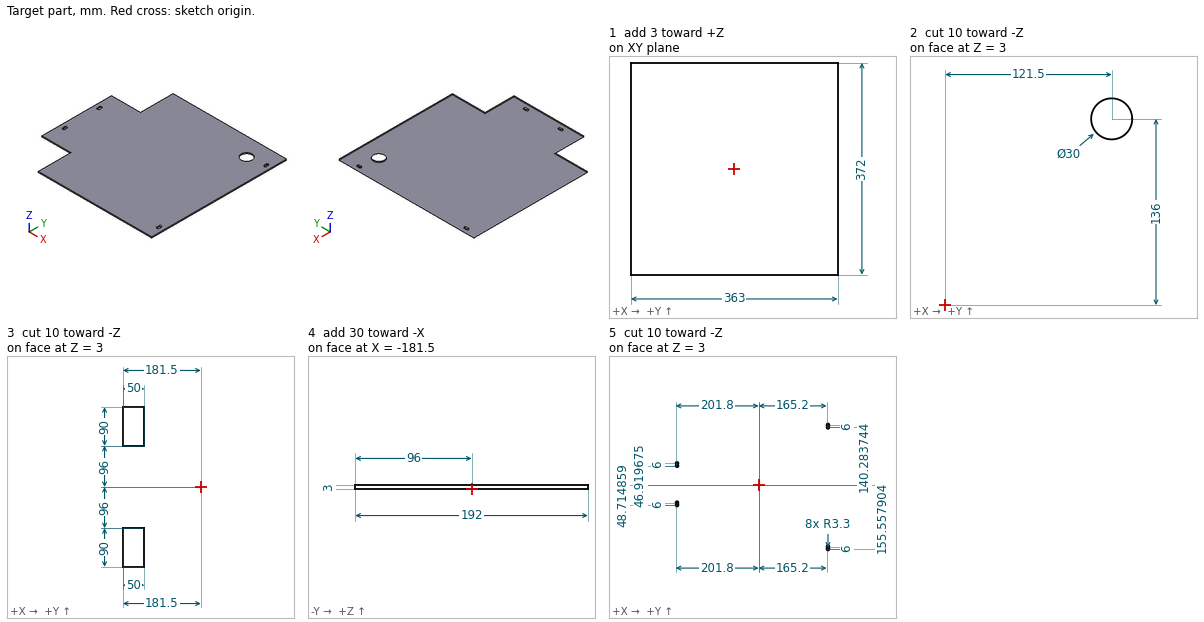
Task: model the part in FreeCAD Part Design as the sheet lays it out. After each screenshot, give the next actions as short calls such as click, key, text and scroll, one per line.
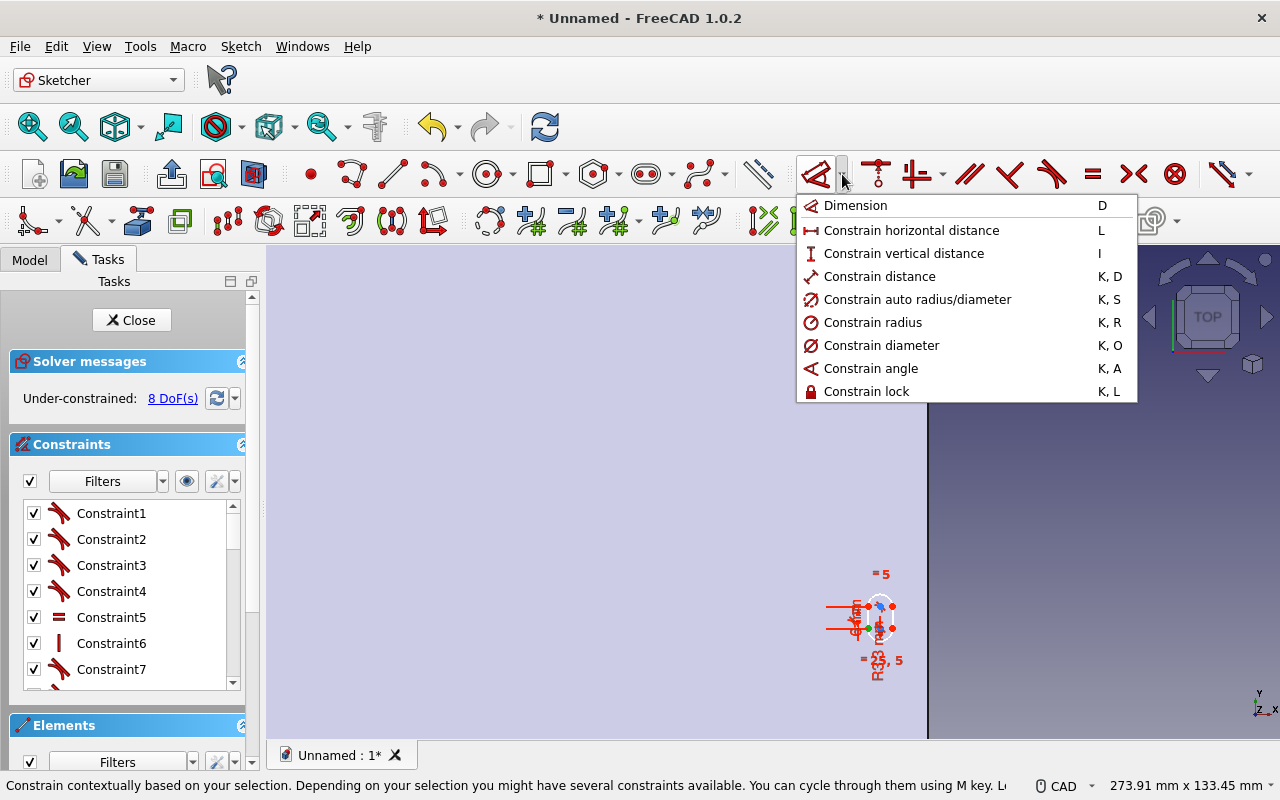
click(967, 230)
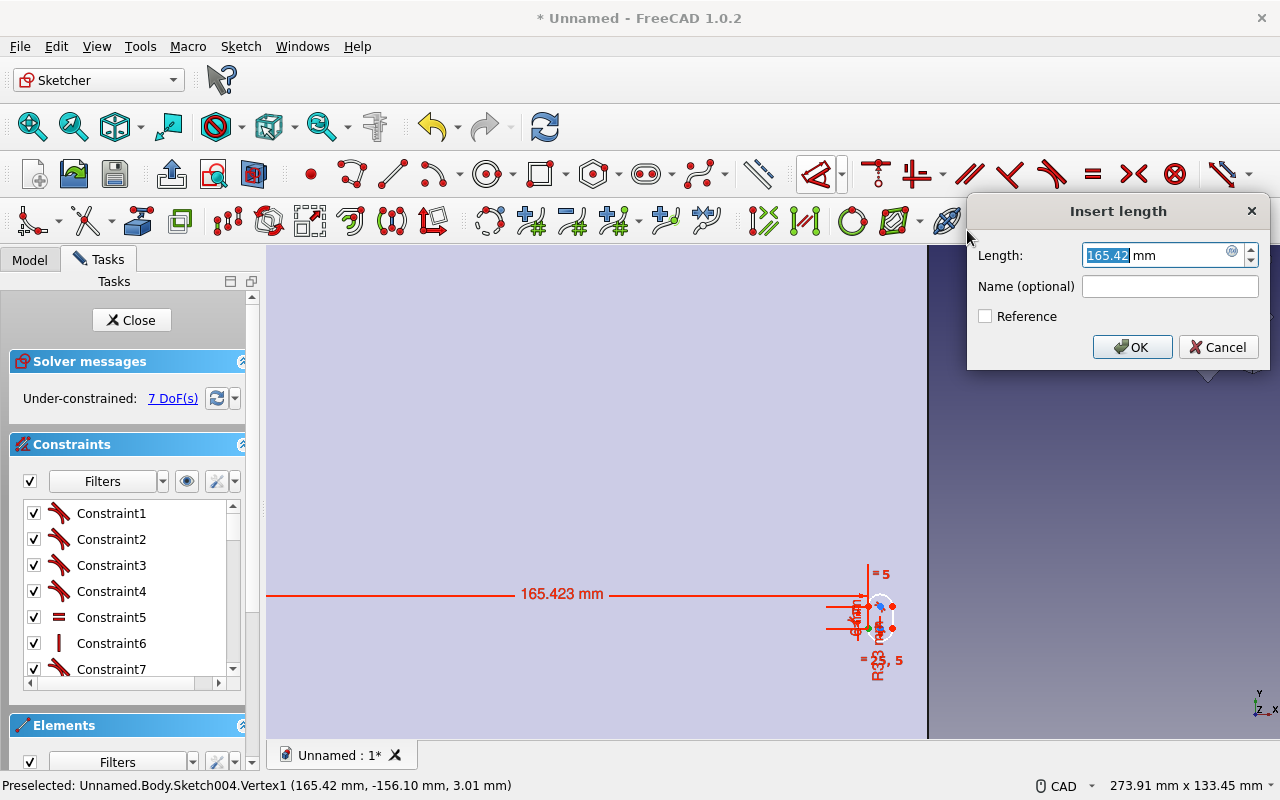
text(165.2)
key(Return)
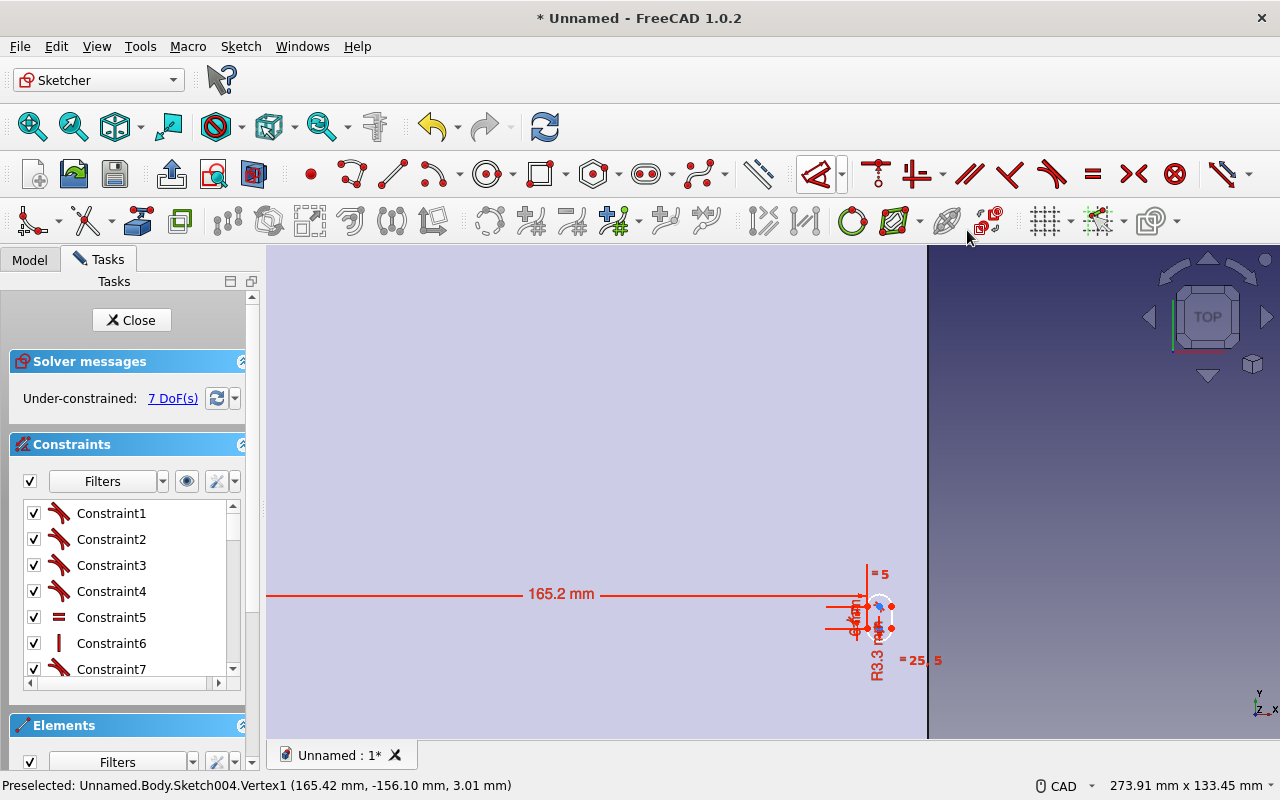
scroll(870, 631, down, 7)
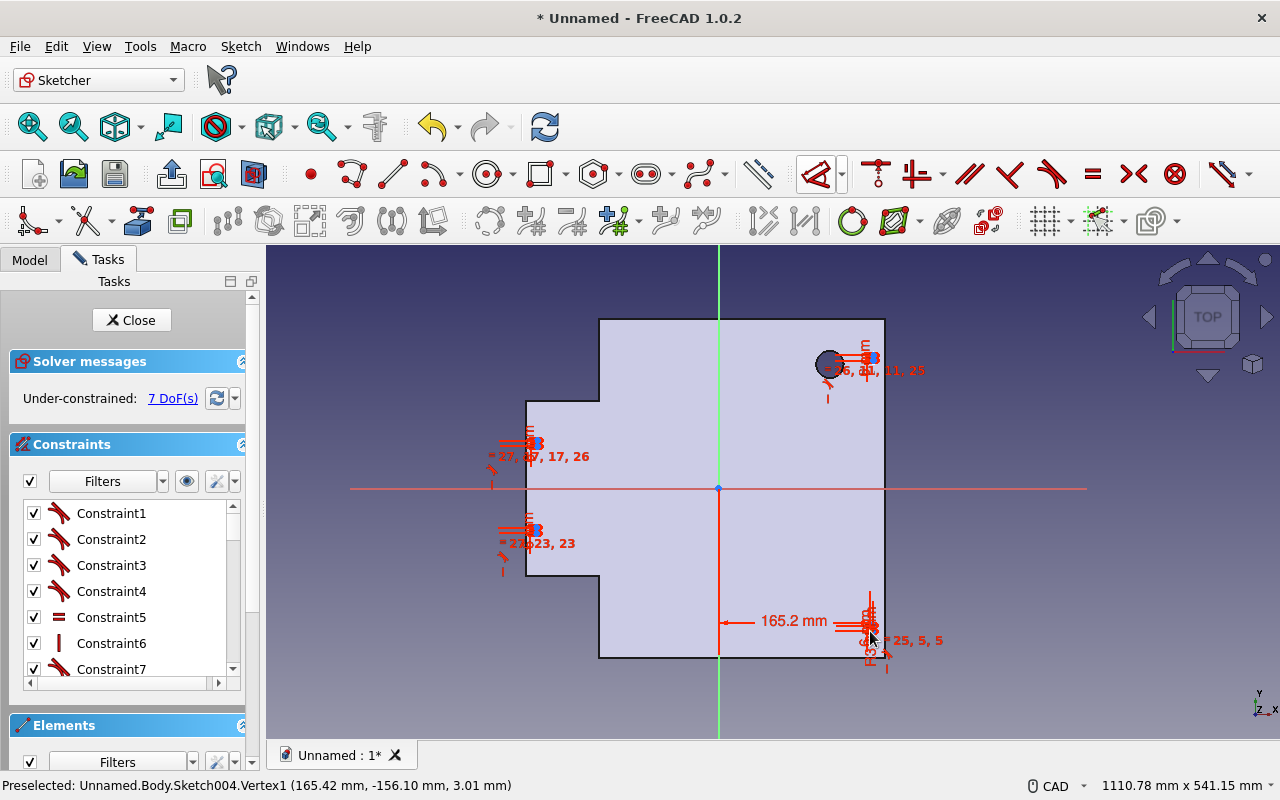
scroll(870, 361, up, 7)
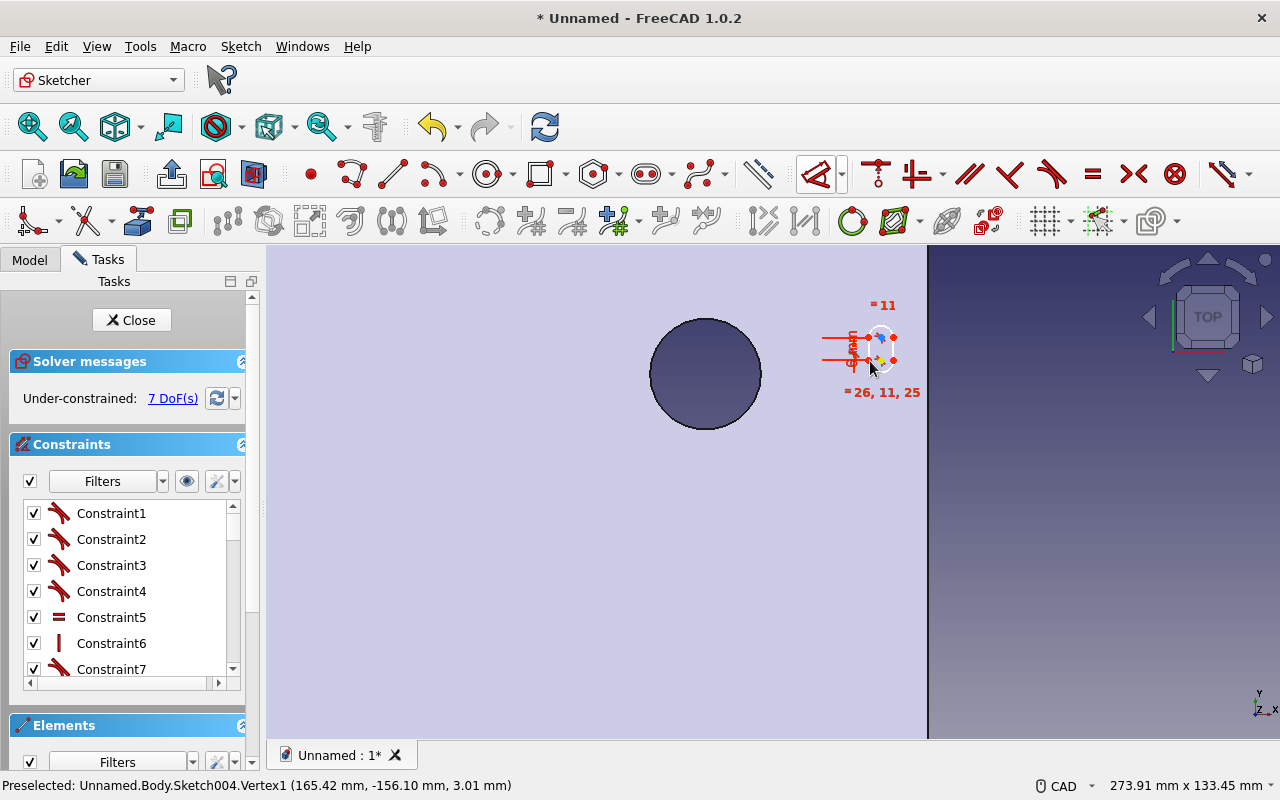
click(869, 360)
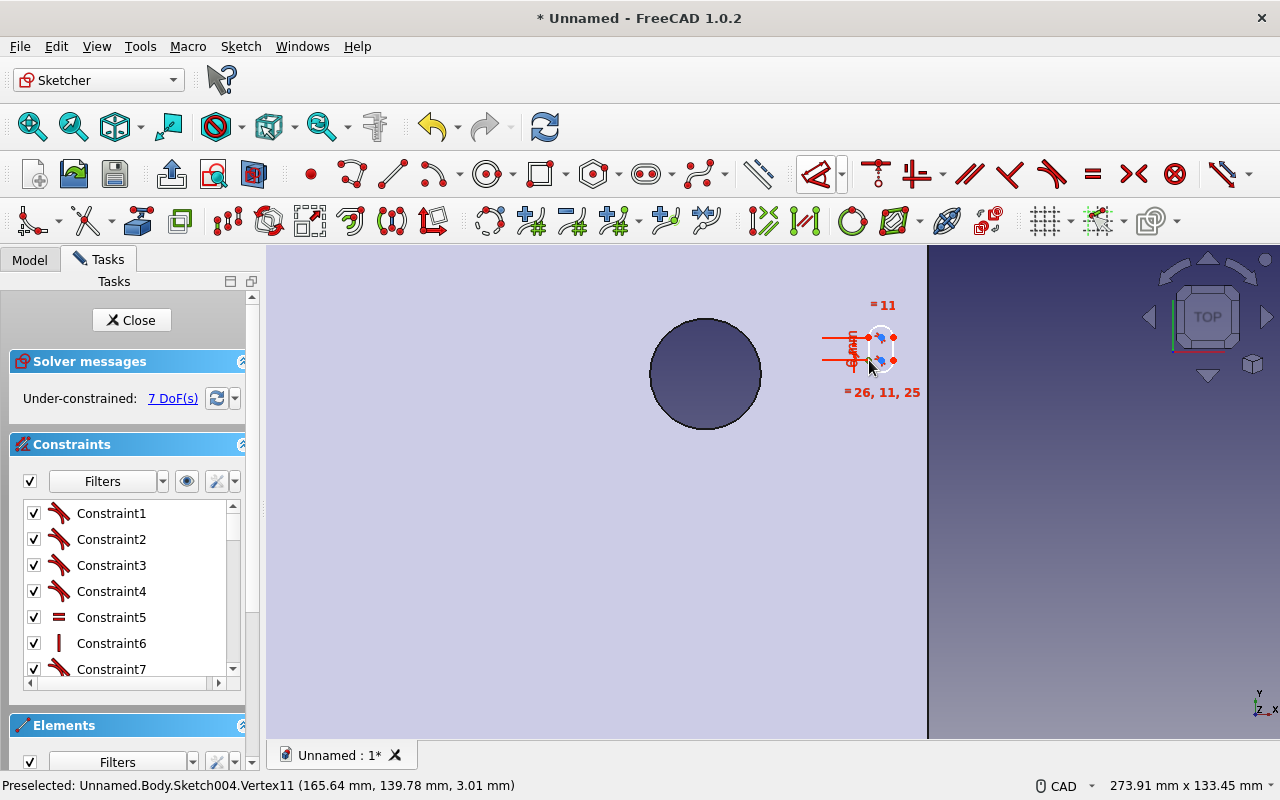
click(842, 174)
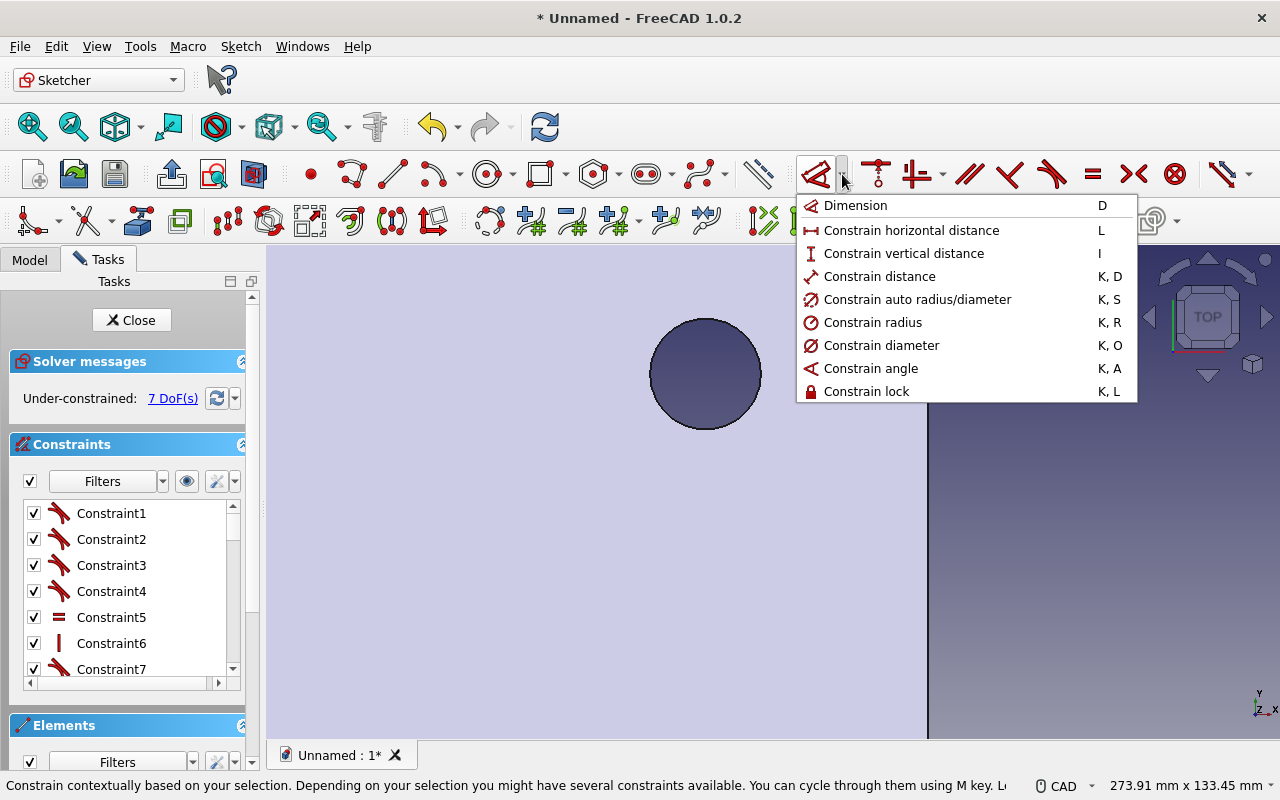
click(967, 230)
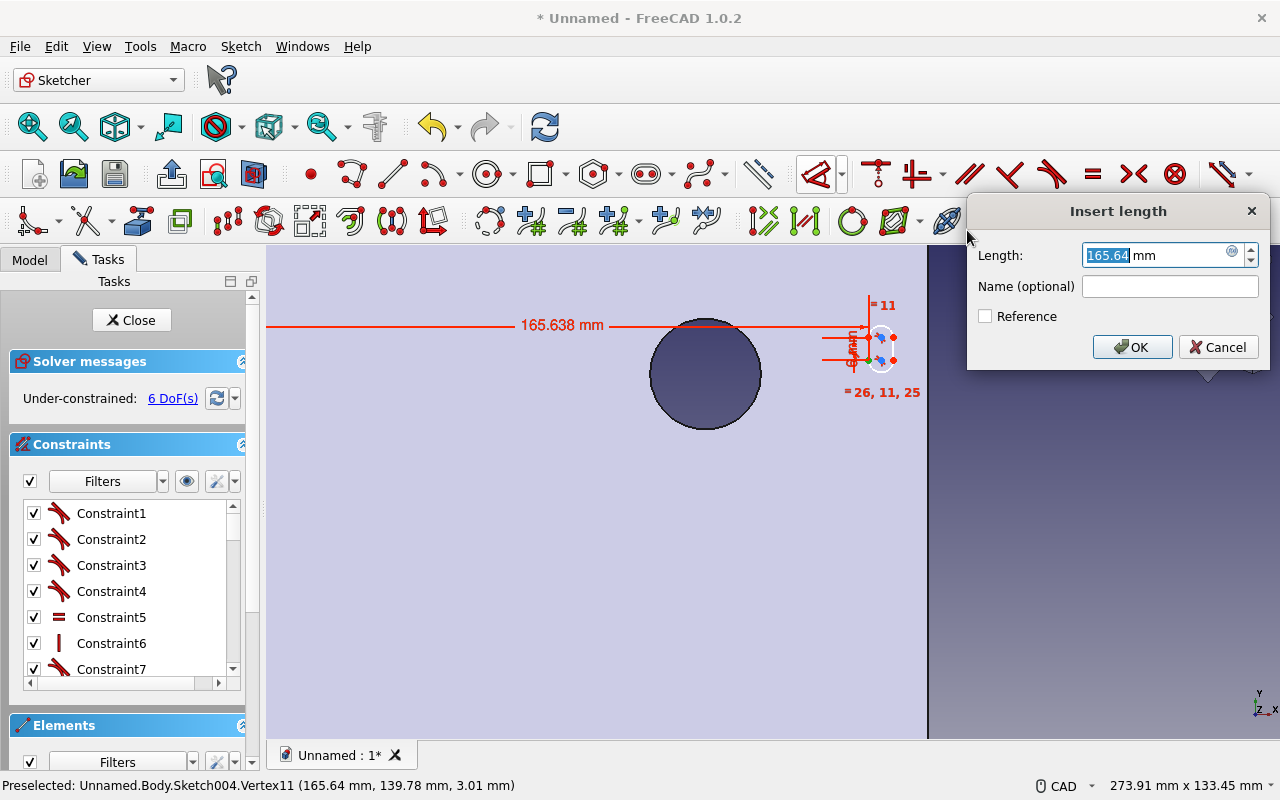
text(165.2)
key(Return)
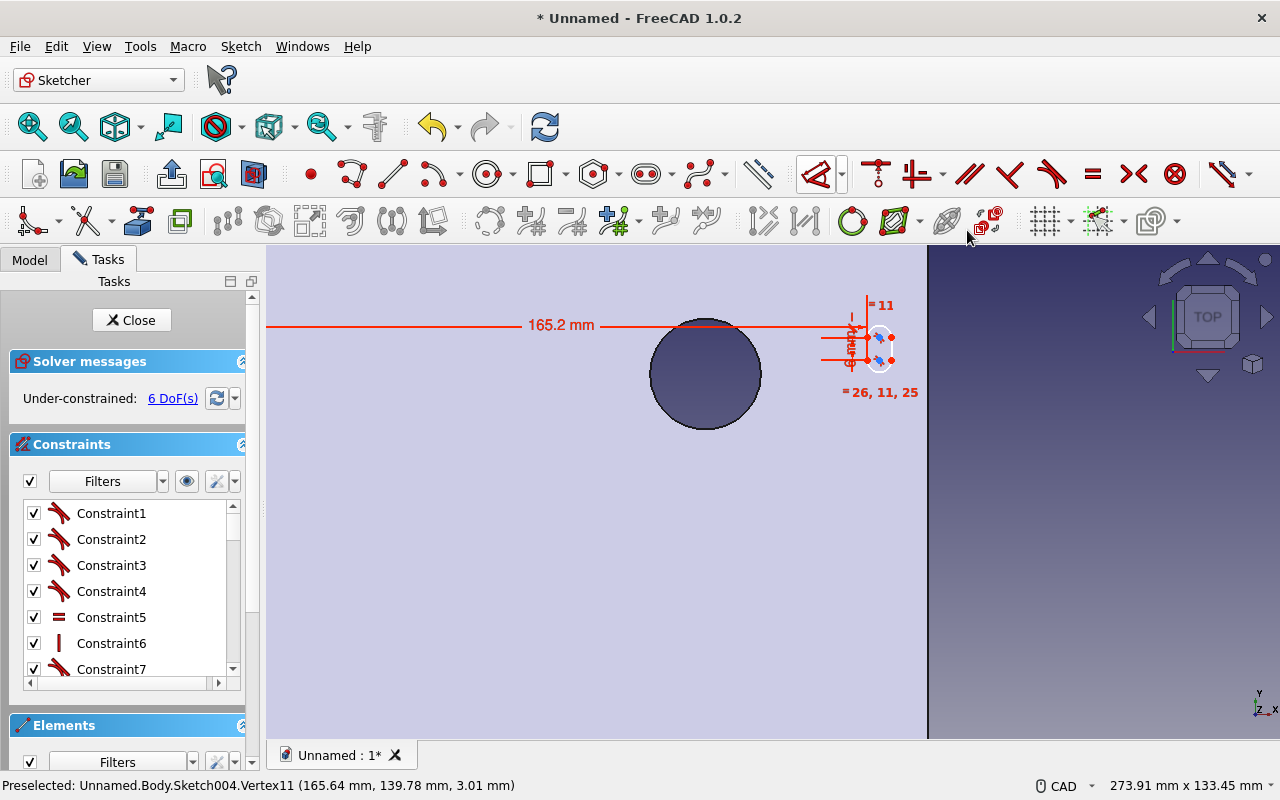
scroll(870, 360, down, 7)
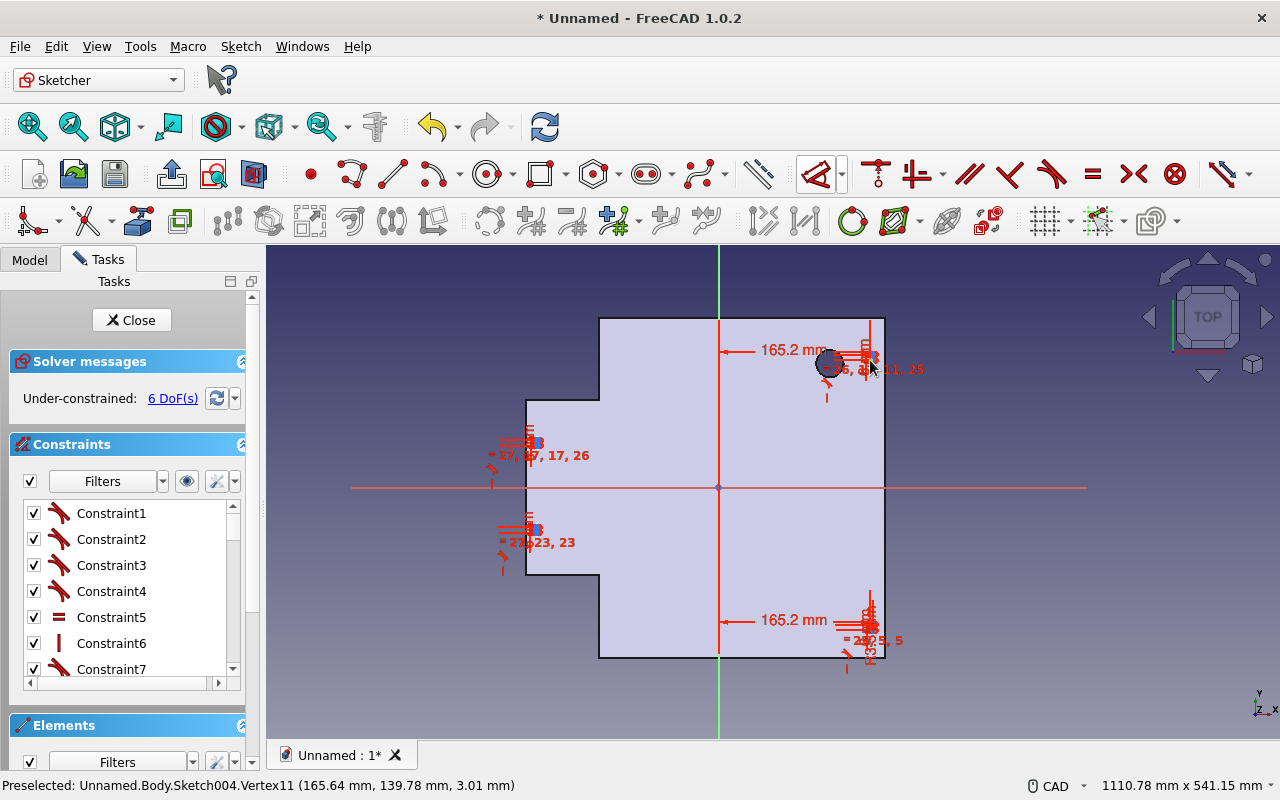
scroll(535, 446, up, 7)